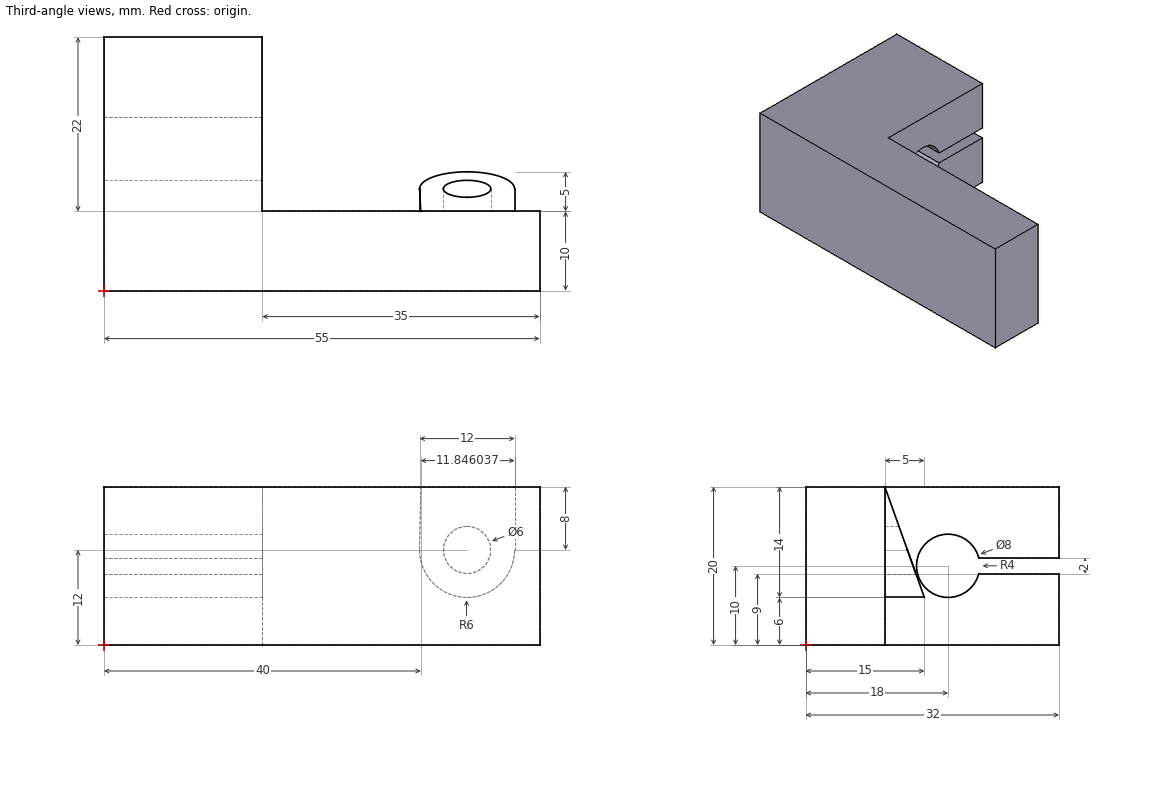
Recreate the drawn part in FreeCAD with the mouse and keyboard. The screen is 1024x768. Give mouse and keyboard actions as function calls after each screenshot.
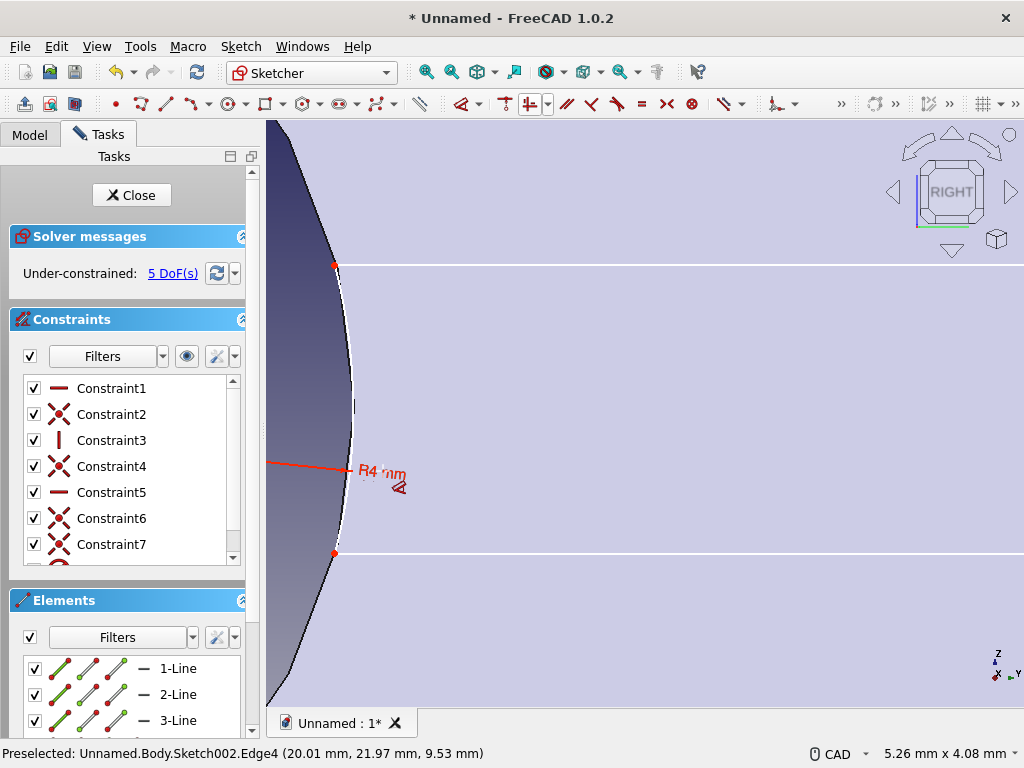
scroll(366, 417, down, 6)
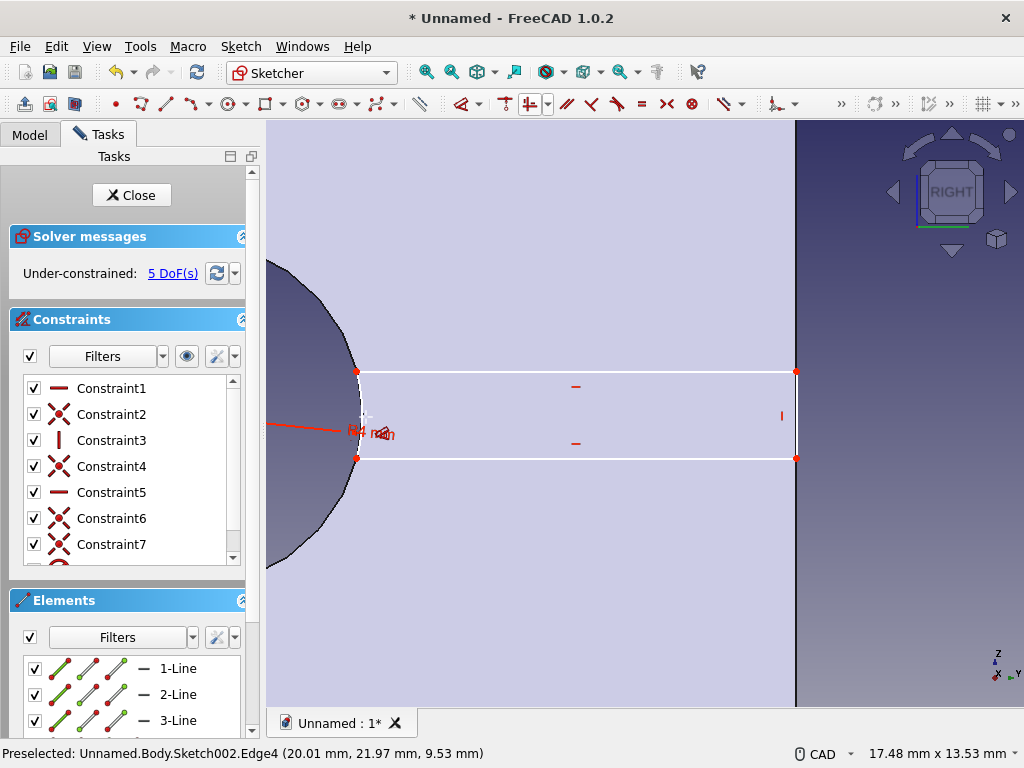
click(797, 432)
click(831, 415)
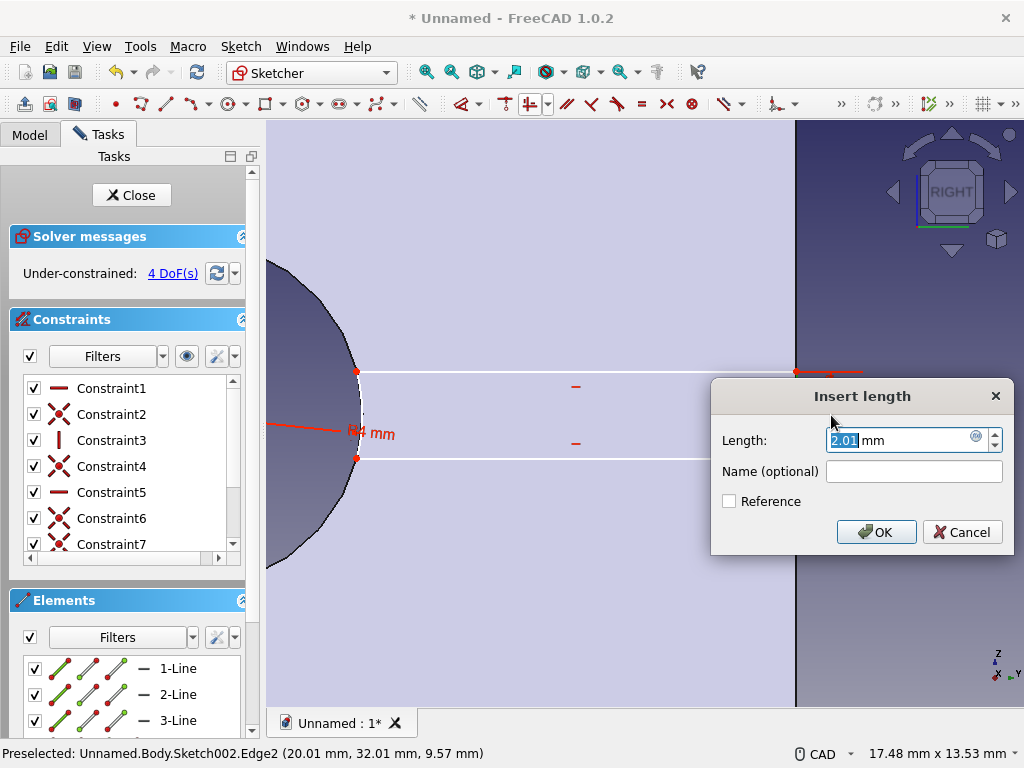
text(2)
key(Return)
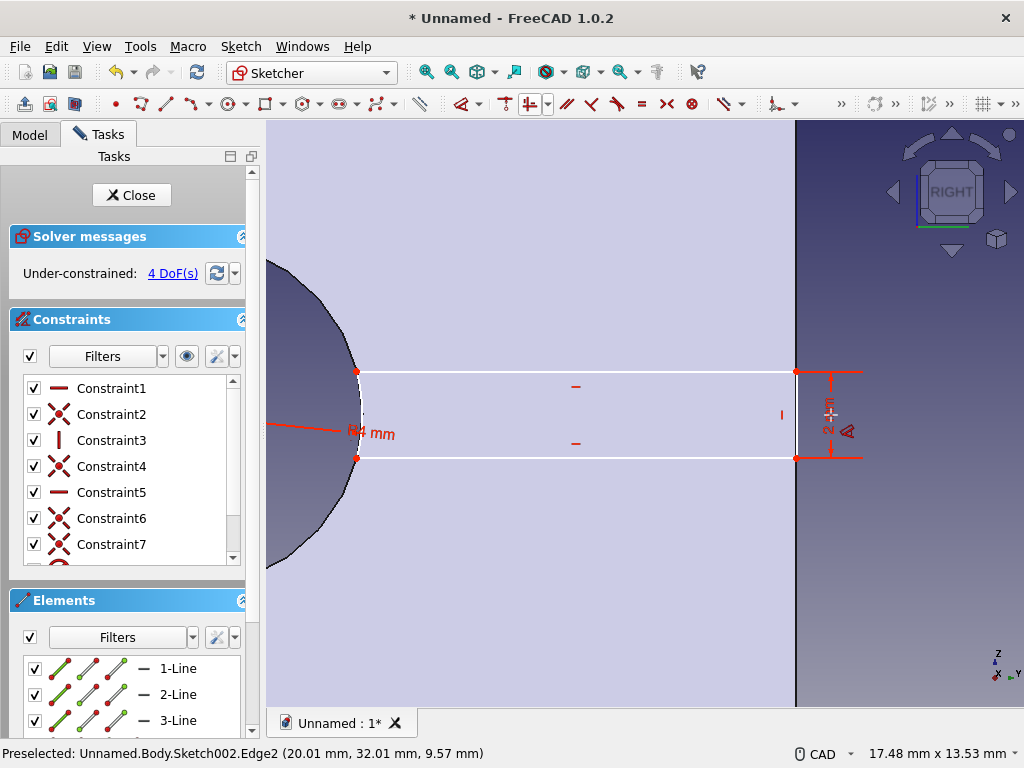
click(357, 458)
click(391, 569)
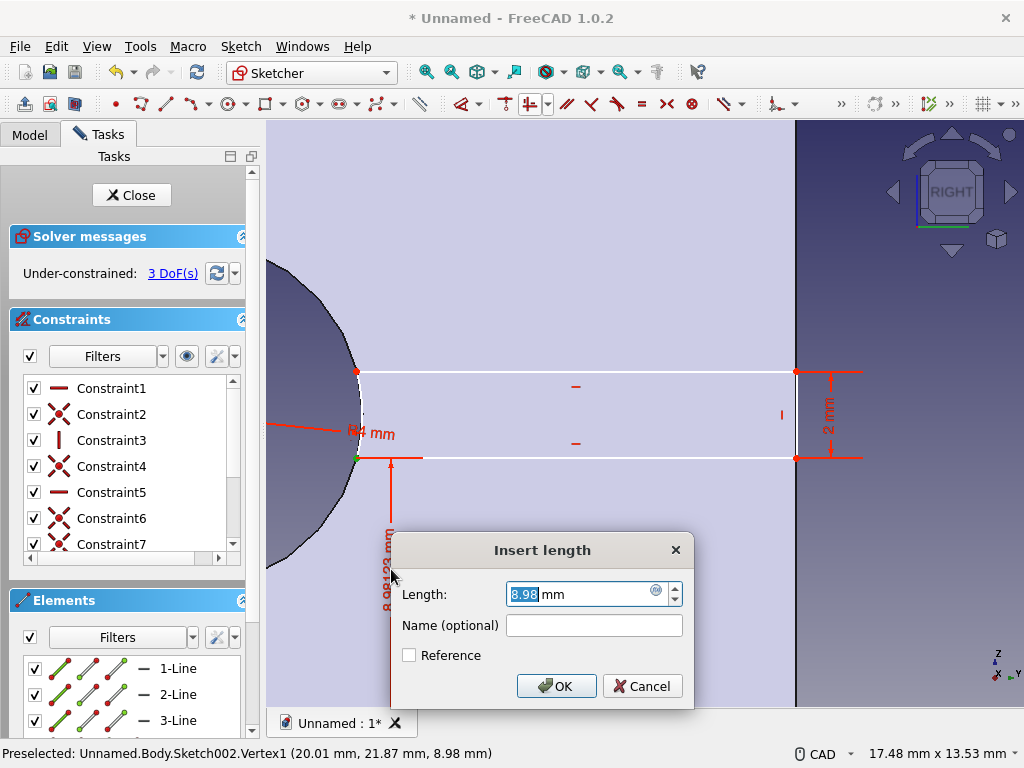
text(9)
key(Return)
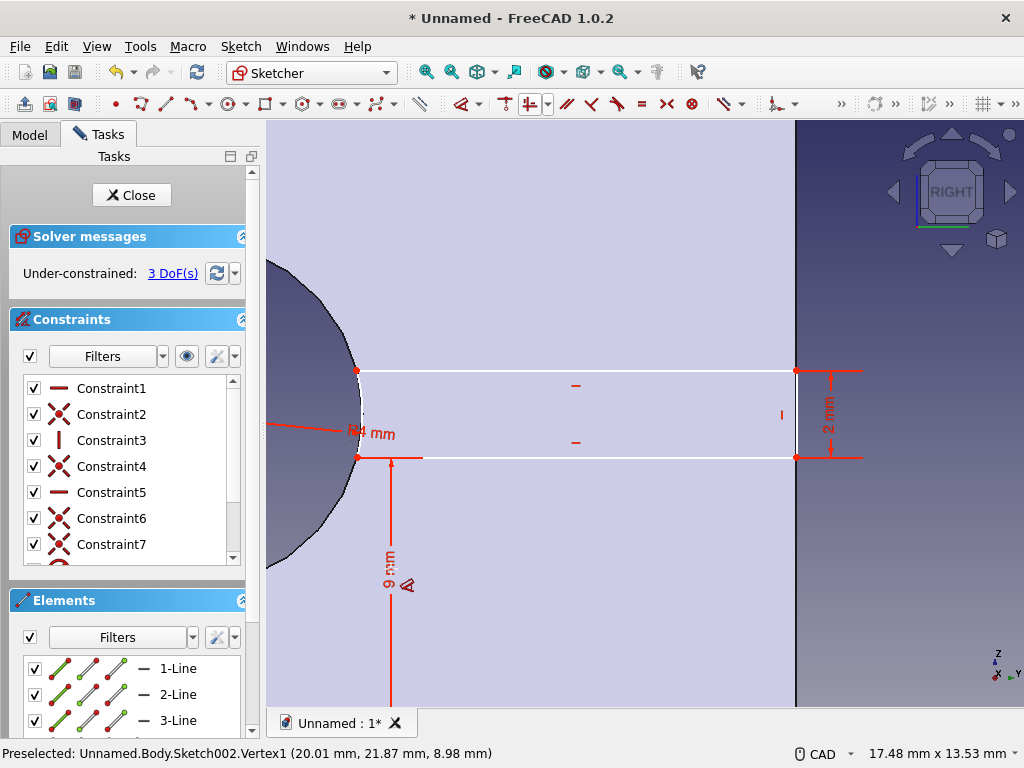
click(797, 458)
click(545, 424)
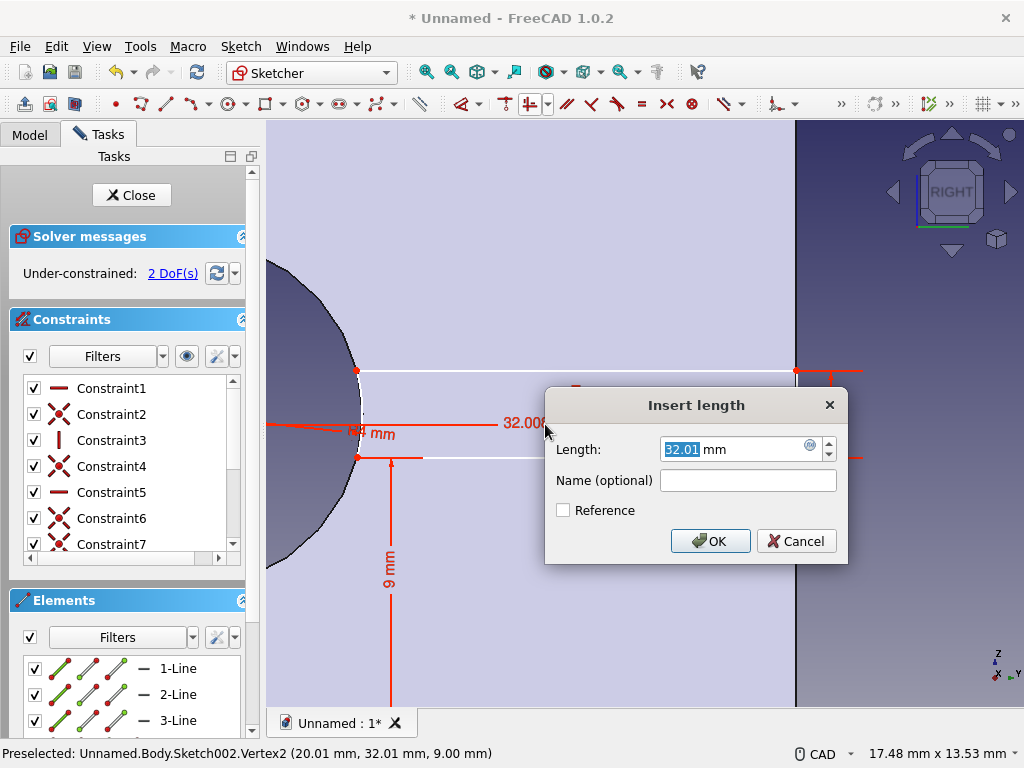
text(32)
key(Return)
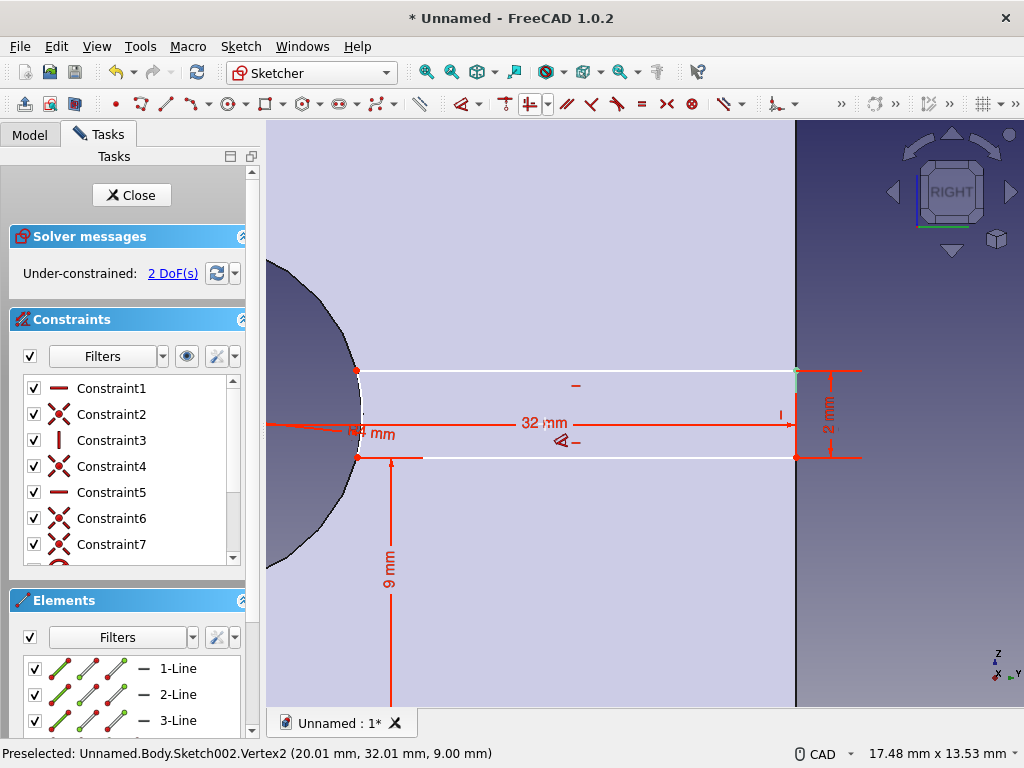
scroll(747, 412, down, 2)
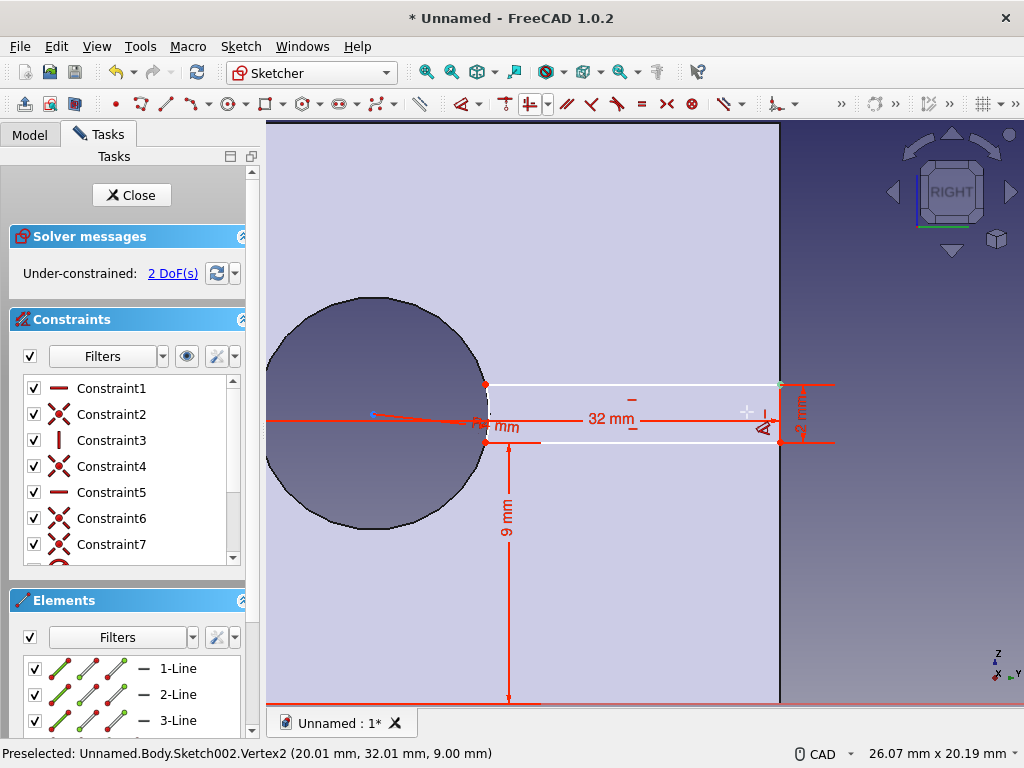
click(373, 414)
click(334, 380)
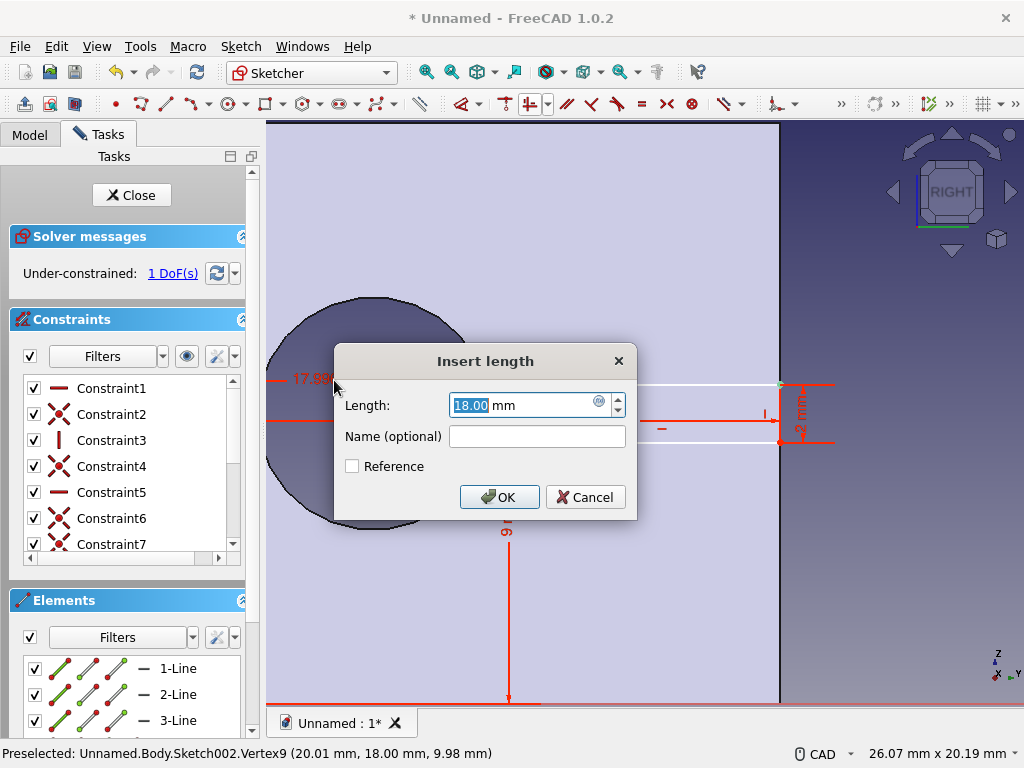
text(18)
key(Return)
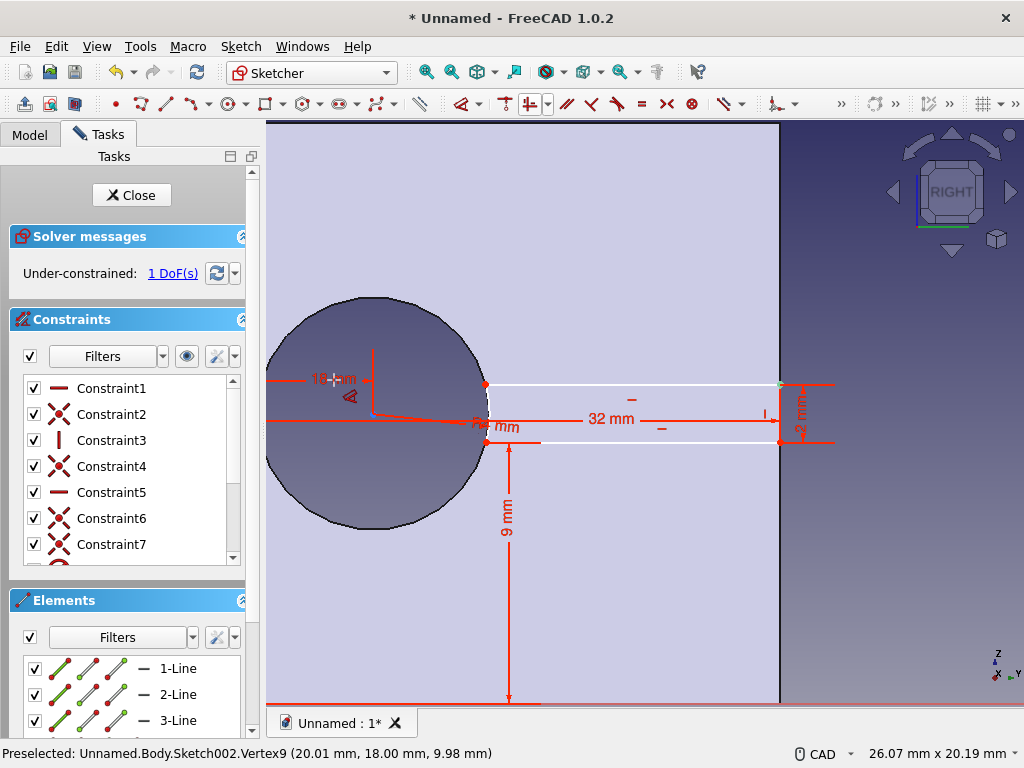
click(373, 414)
click(407, 547)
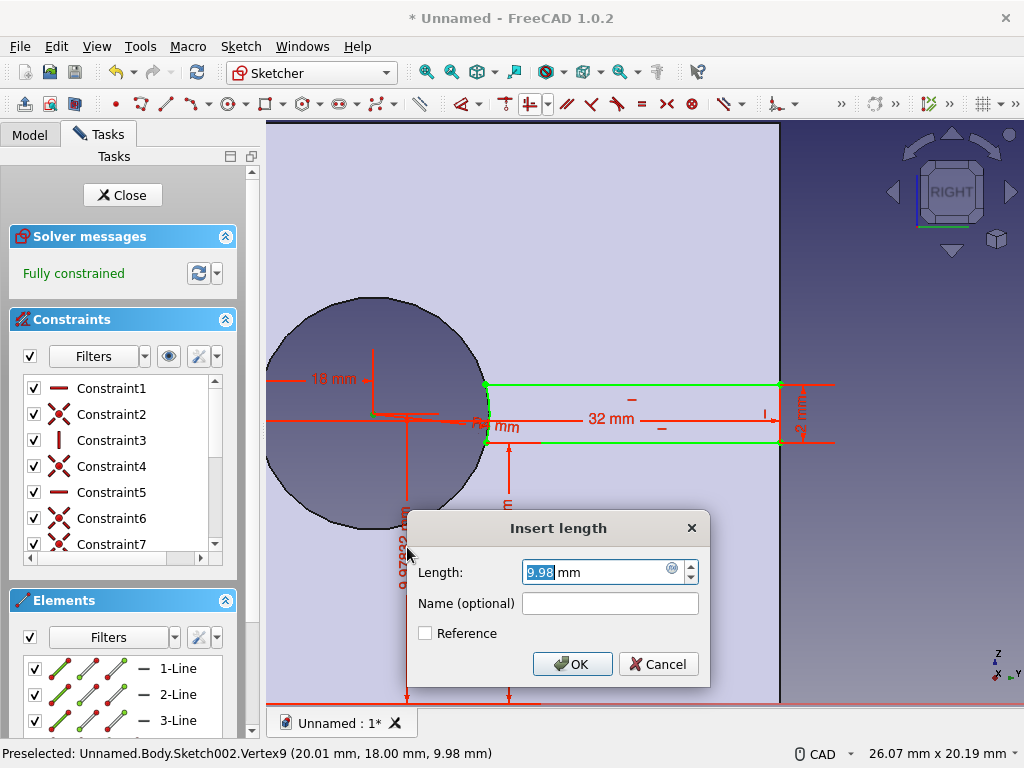
text(10)
key(Return)
key(Escape)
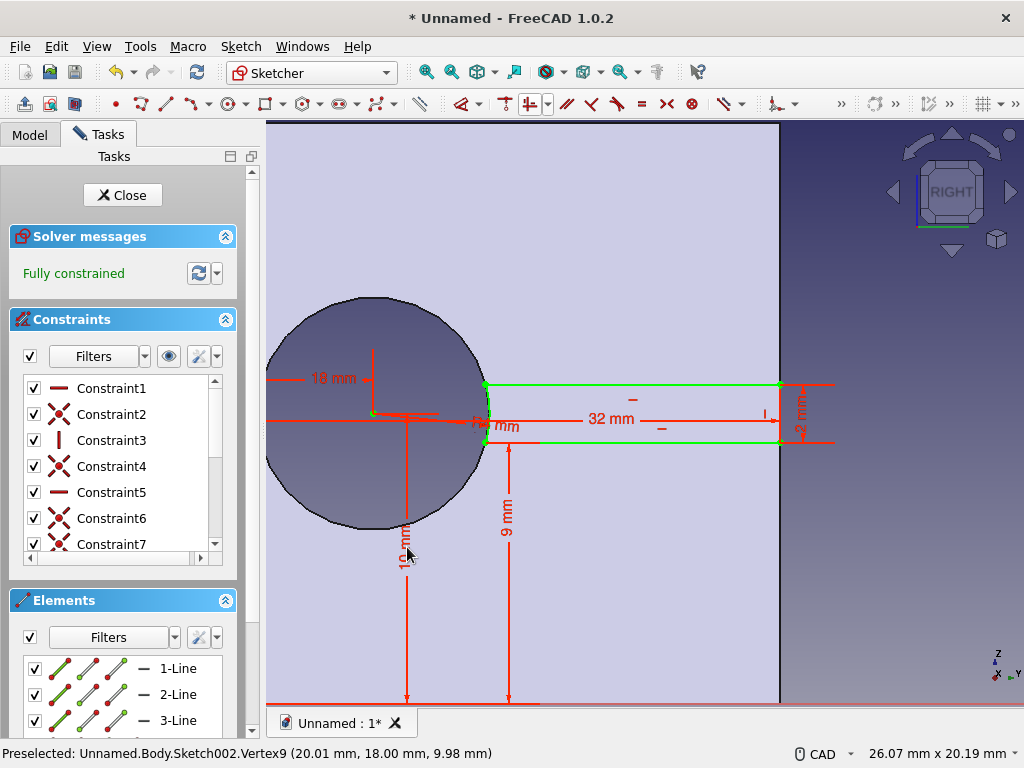
click(123, 195)